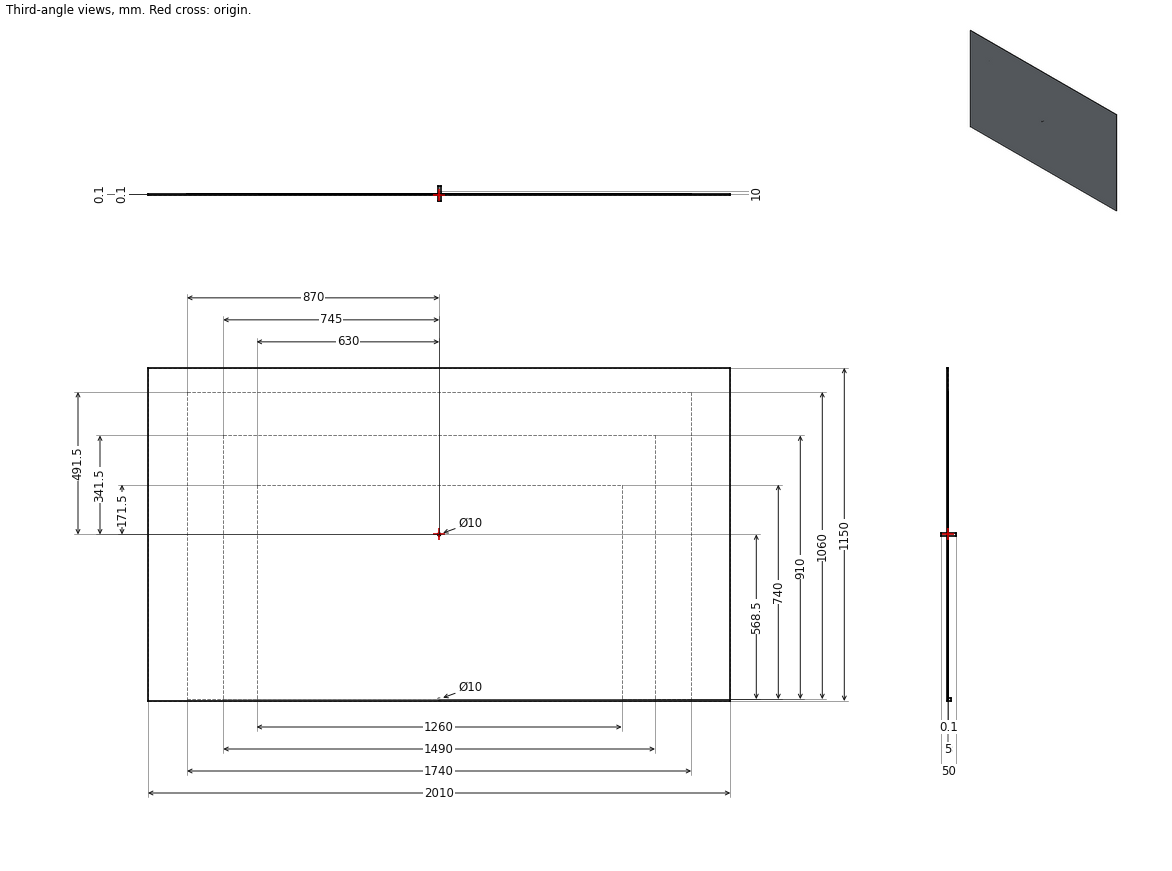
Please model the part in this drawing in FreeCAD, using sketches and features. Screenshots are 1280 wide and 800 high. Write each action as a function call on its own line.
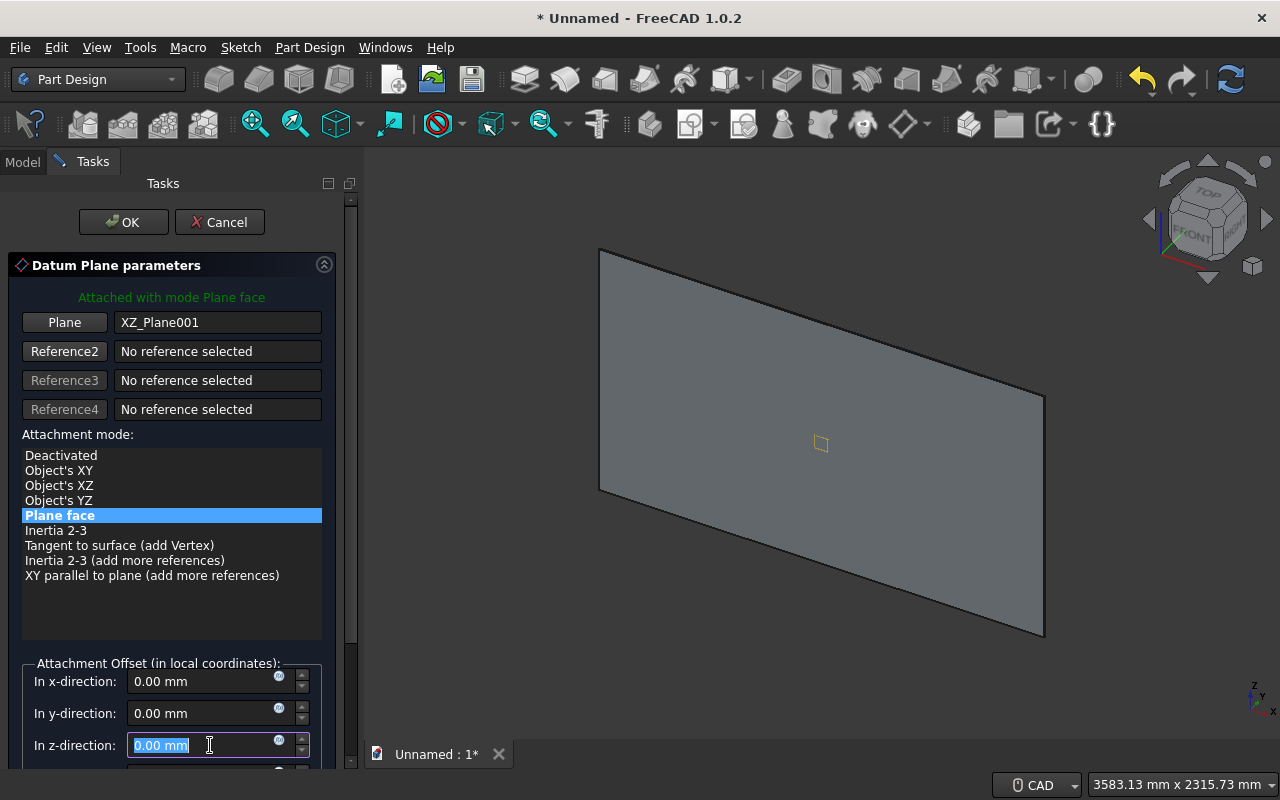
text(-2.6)
key(Tab)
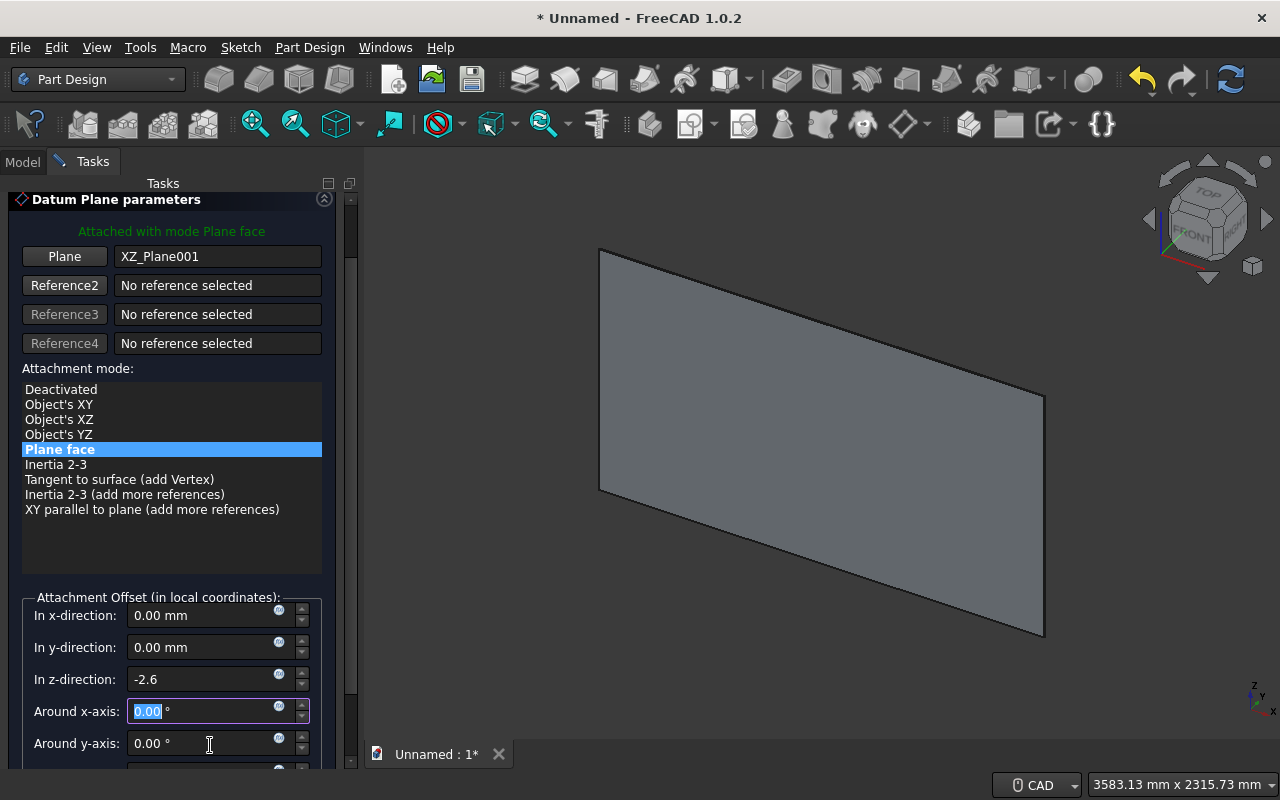
scroll(351, 480, up, 2)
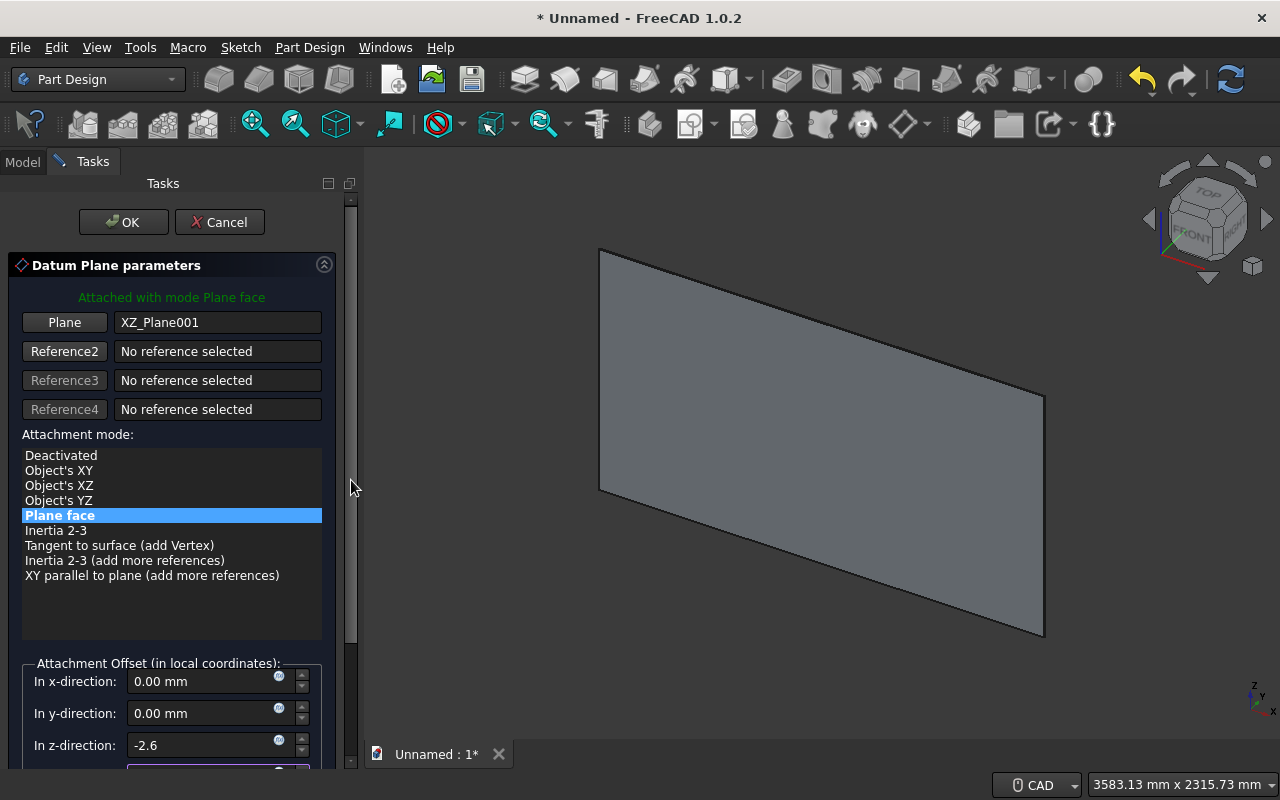
click(124, 222)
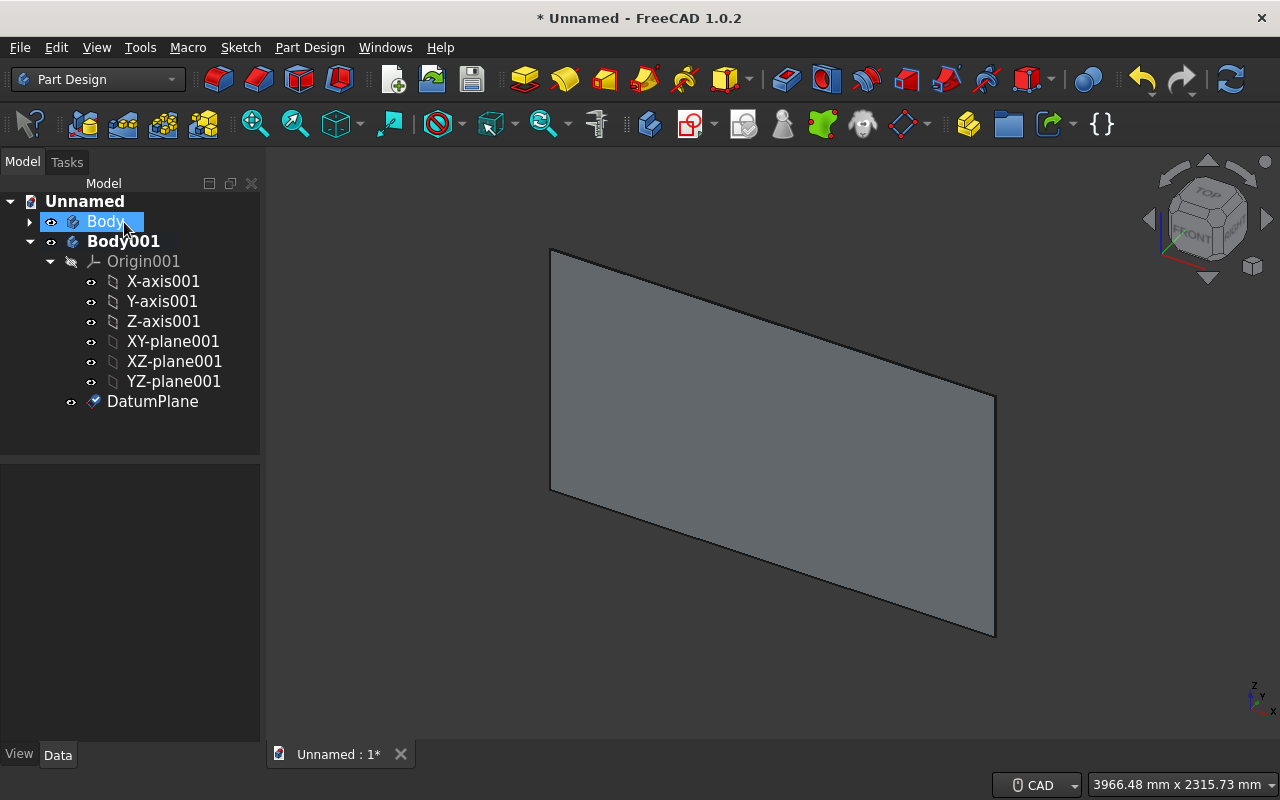
click(116, 402)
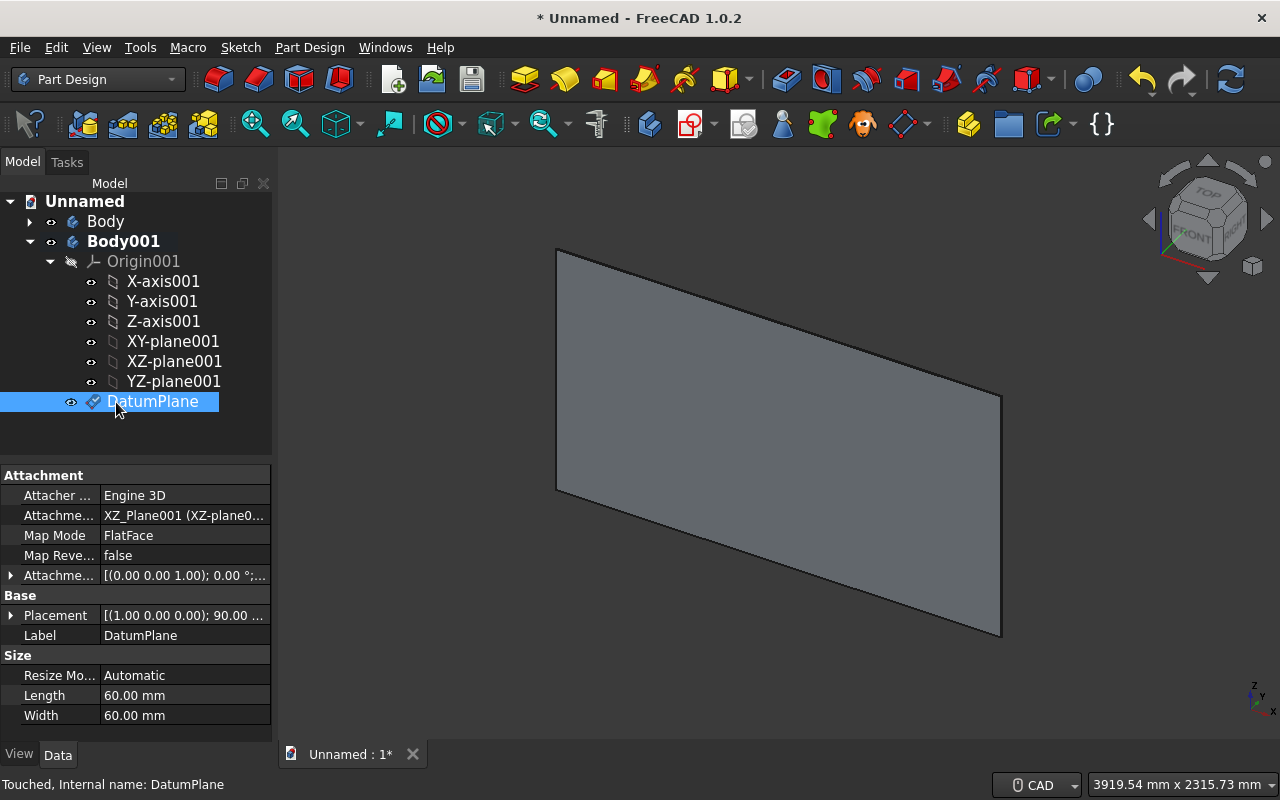
click(690, 124)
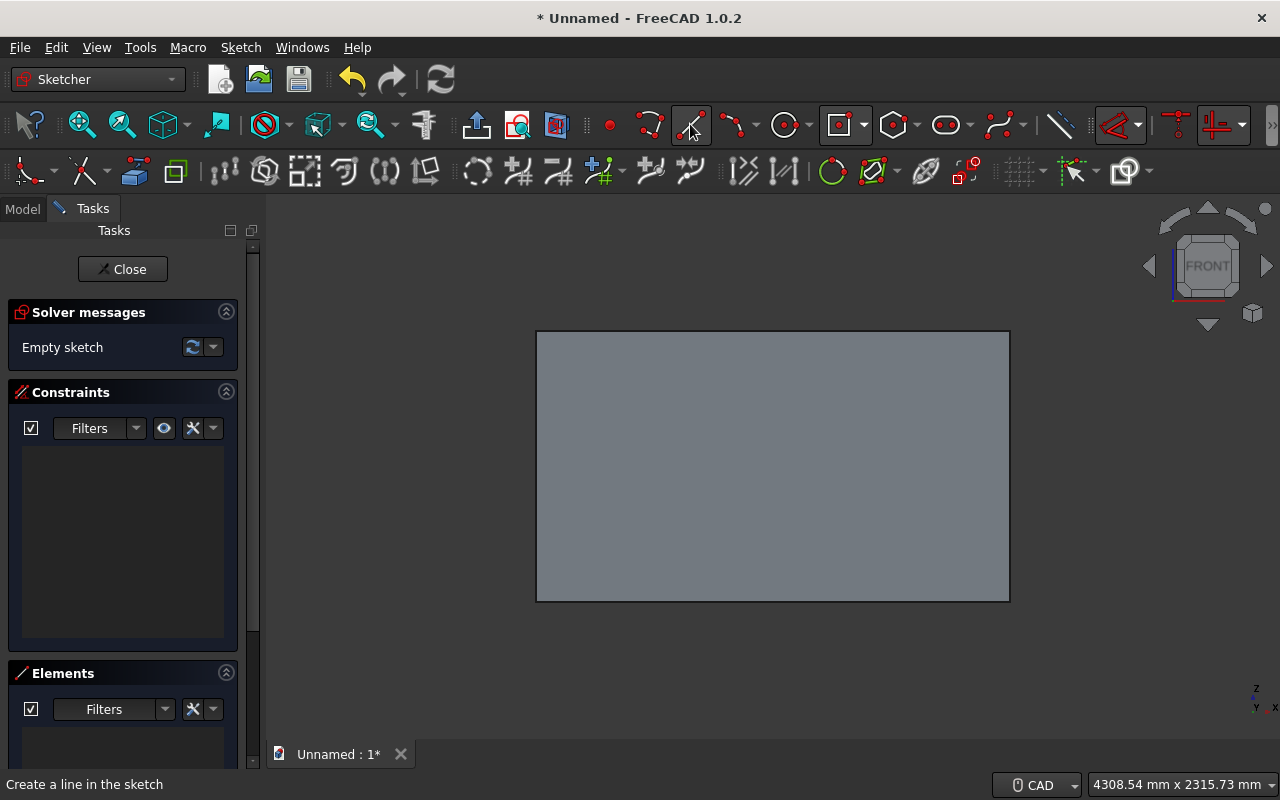
scroll(912, 494, up, 2)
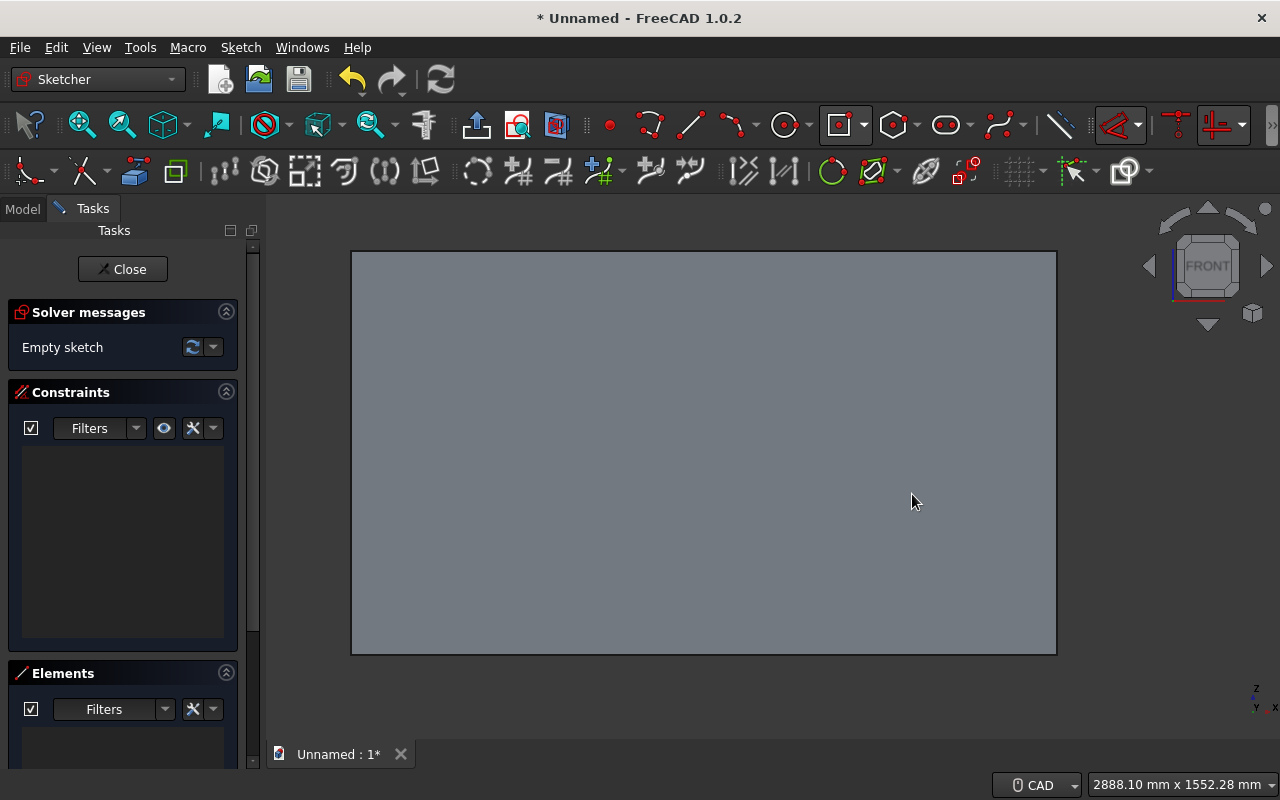
key(g)
key(r)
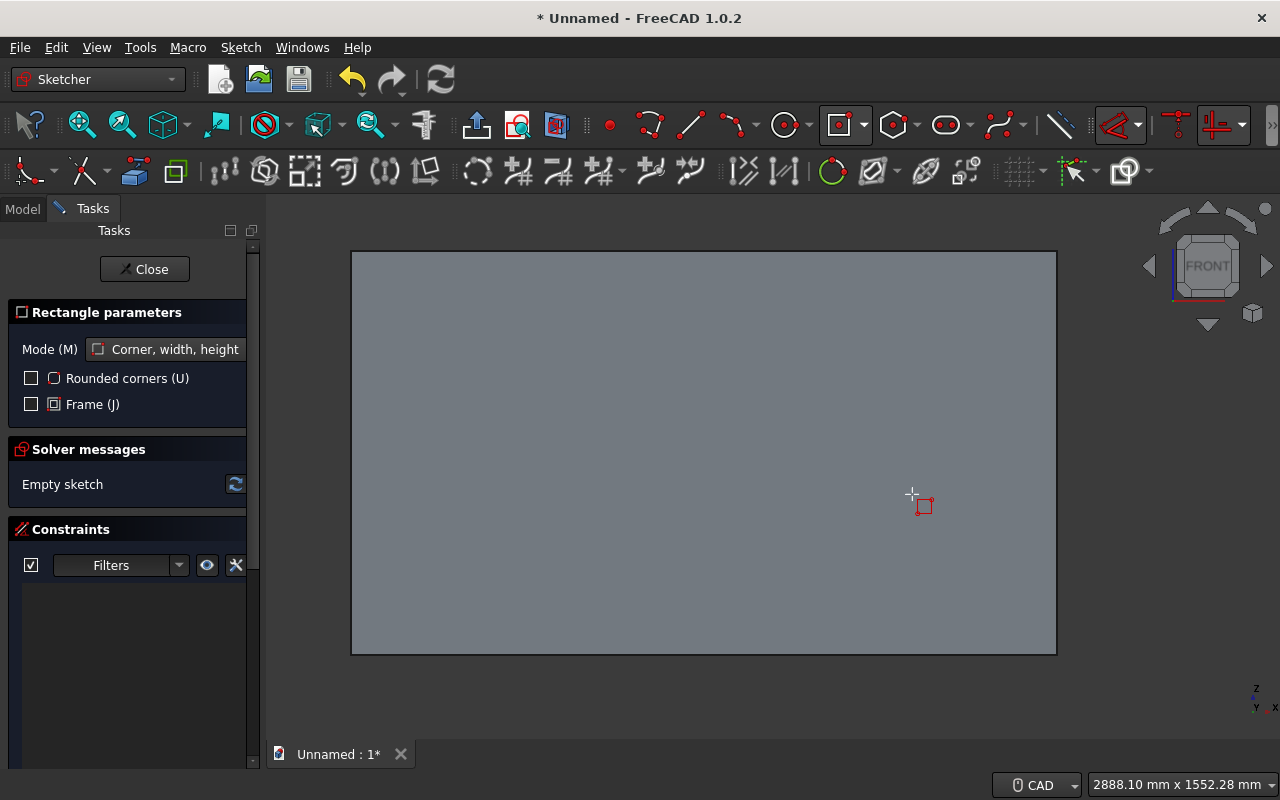
click(399, 280)
move(1010, 652)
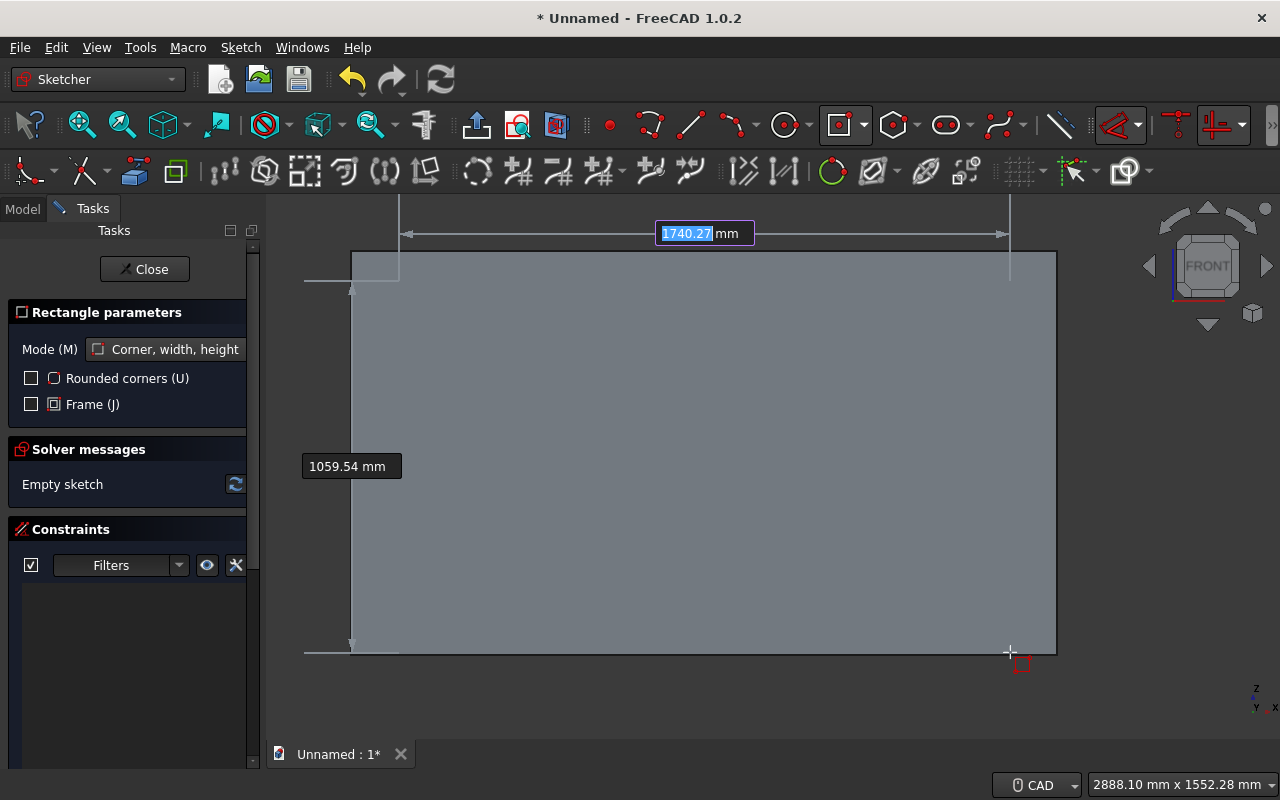
text(1740)
key(Tab)
text(1060)
key(Return)
key(Escape)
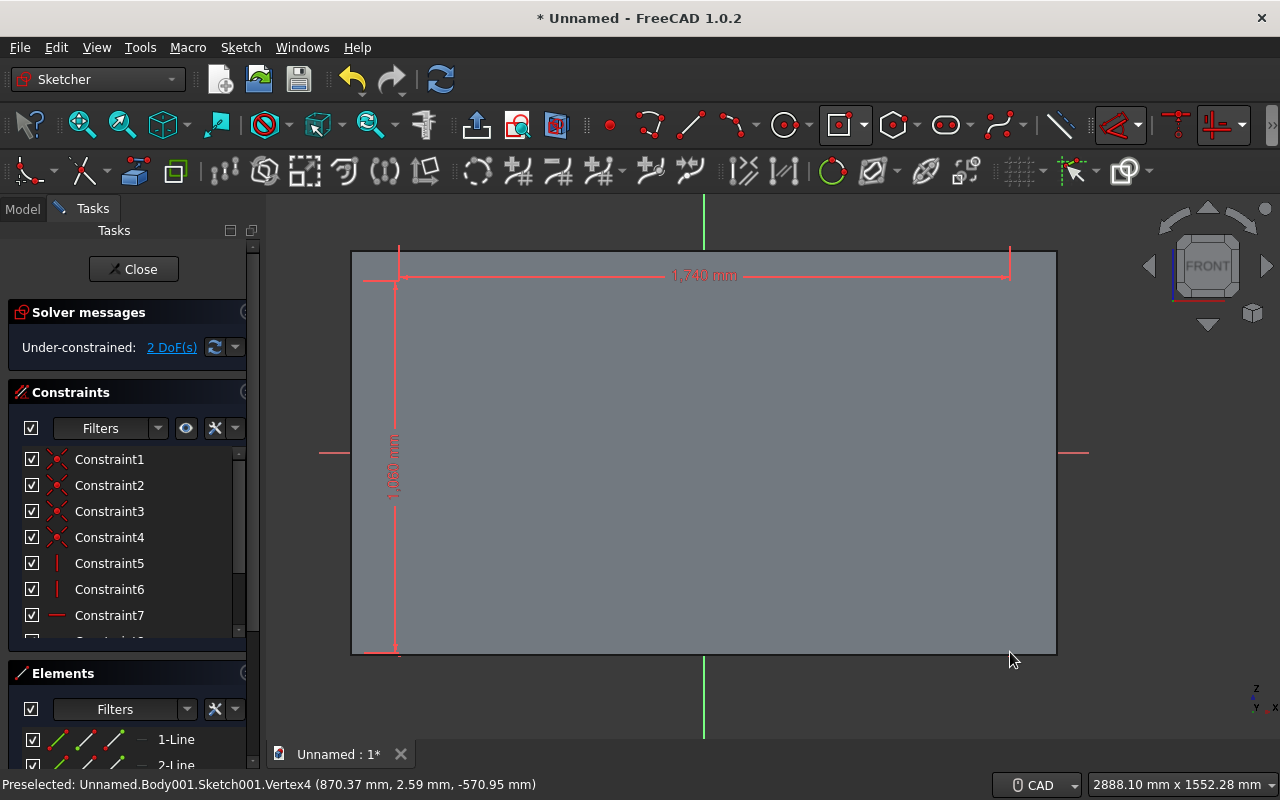
click(1114, 126)